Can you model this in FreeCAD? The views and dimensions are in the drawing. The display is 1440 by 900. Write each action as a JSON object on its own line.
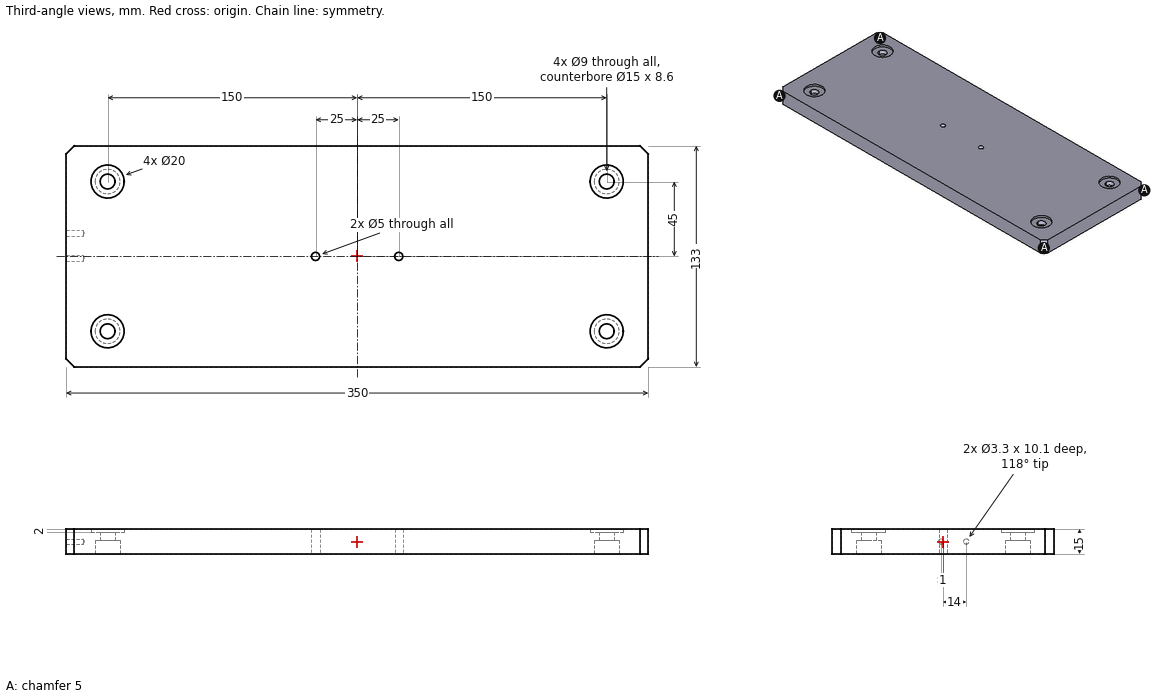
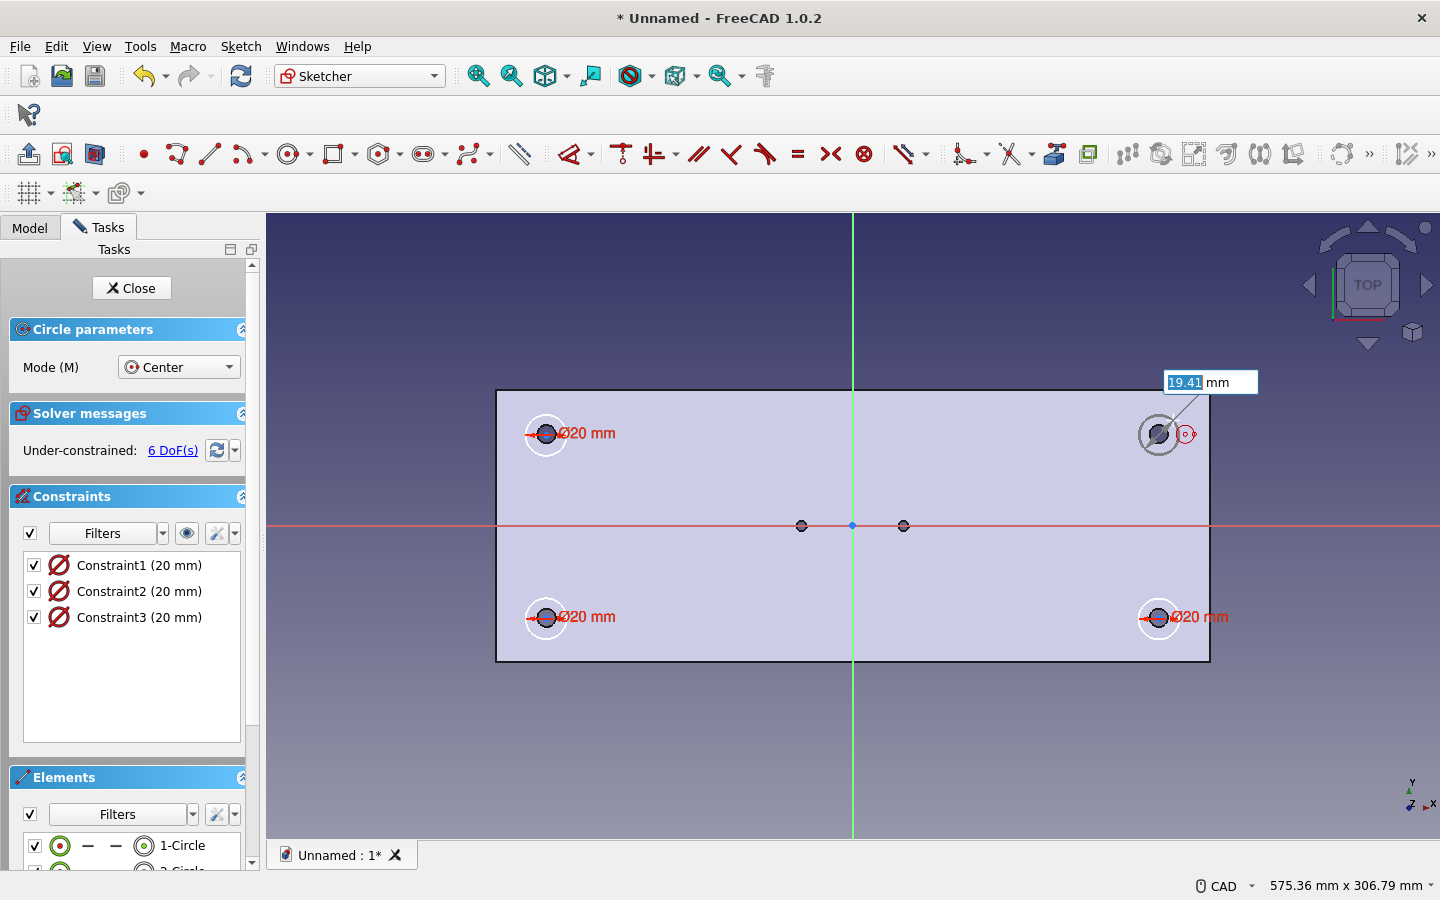
{"action": "type", "text": "20"}
{"action": "key", "text": "Return"}
{"action": "key", "text": "Escape"}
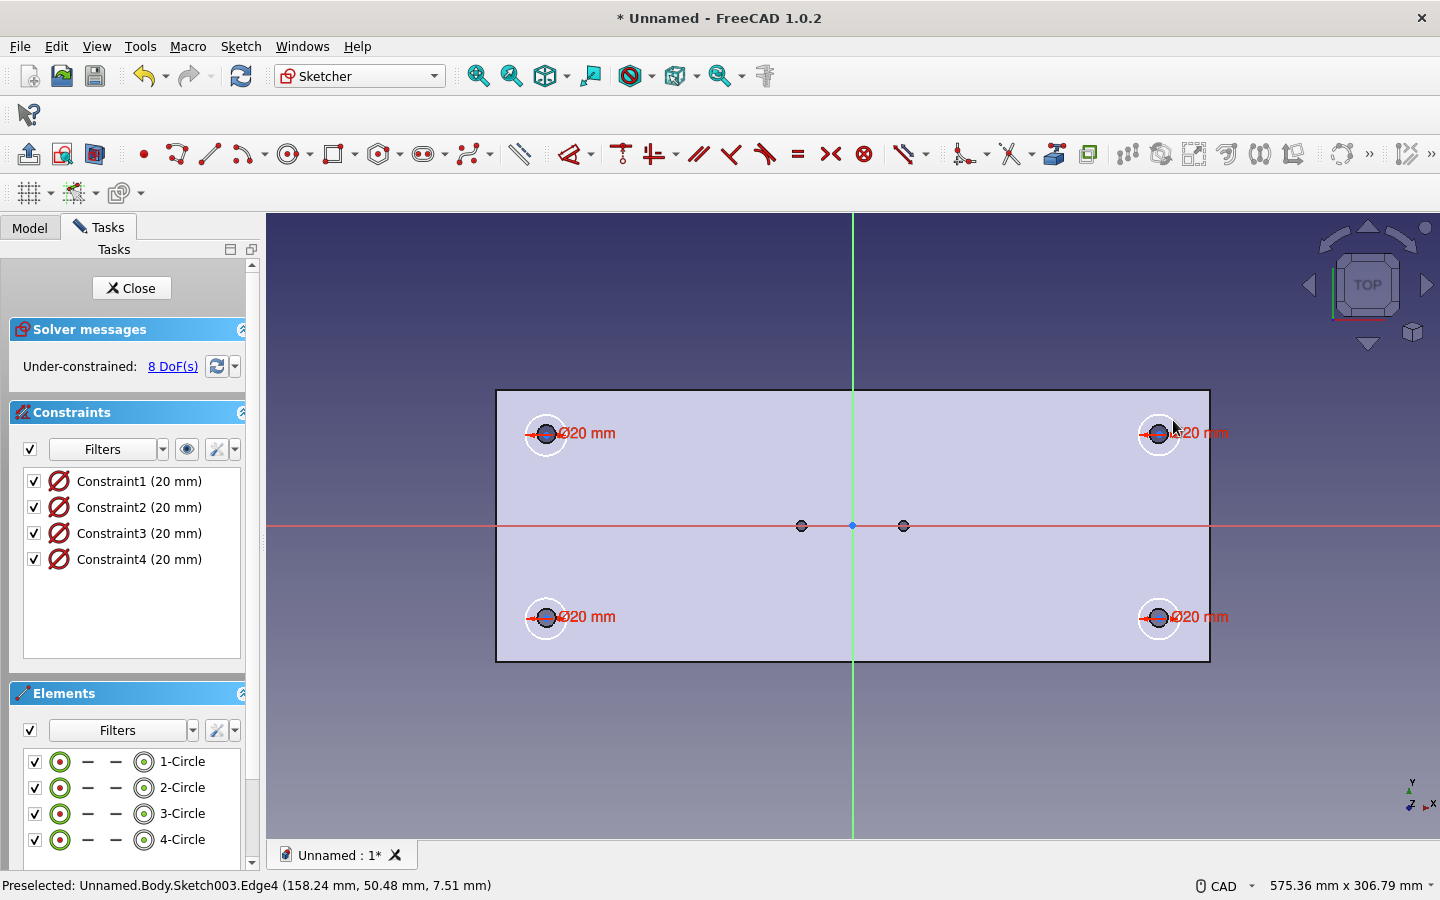
{"action": "left_click", "coordinate": [546, 435]}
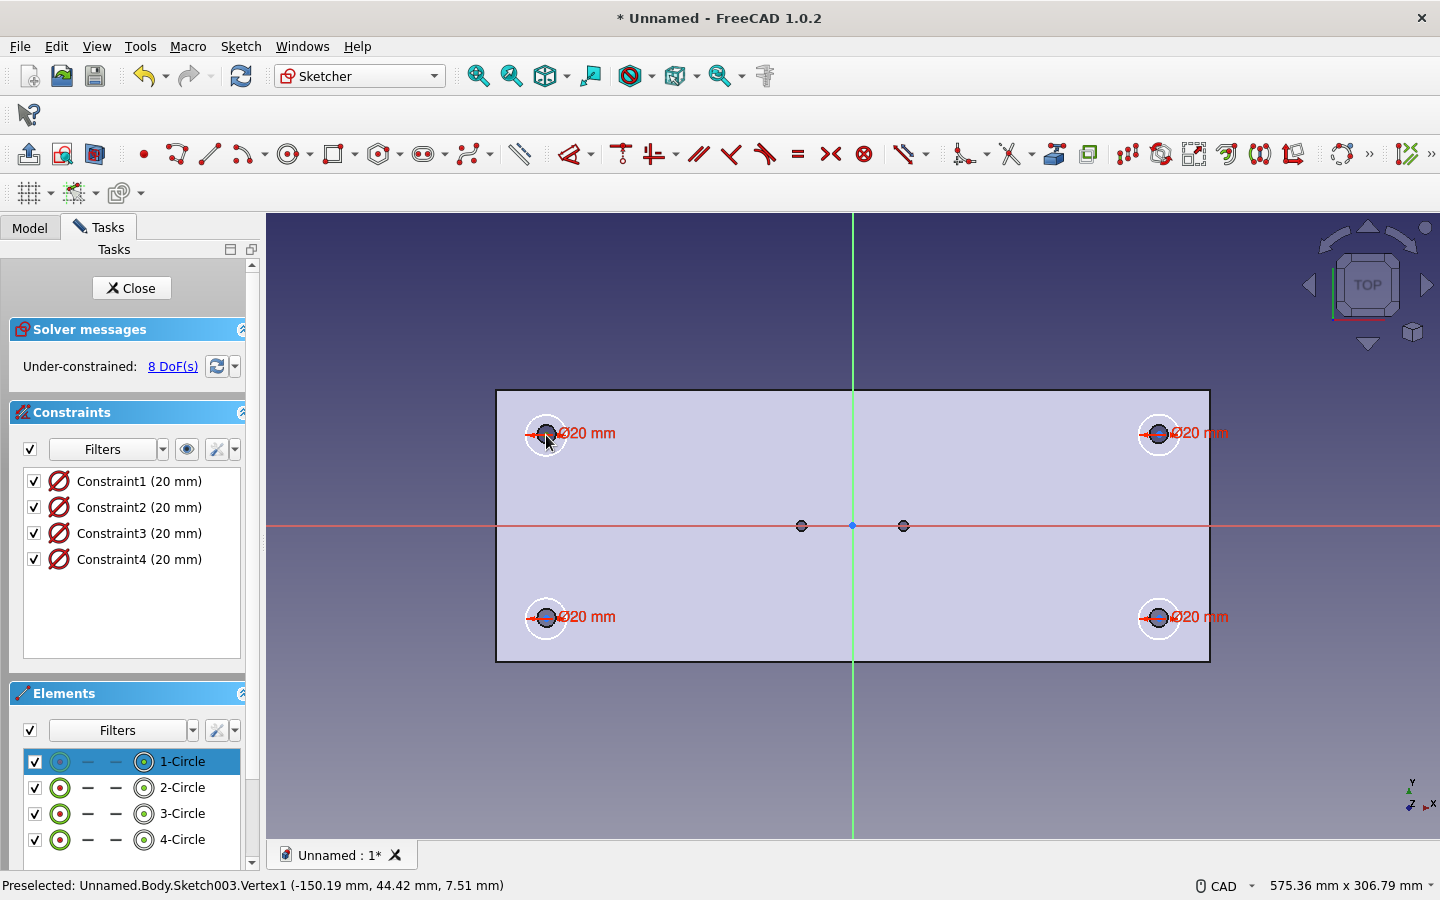
{"action": "left_click", "coordinate": [546, 619]}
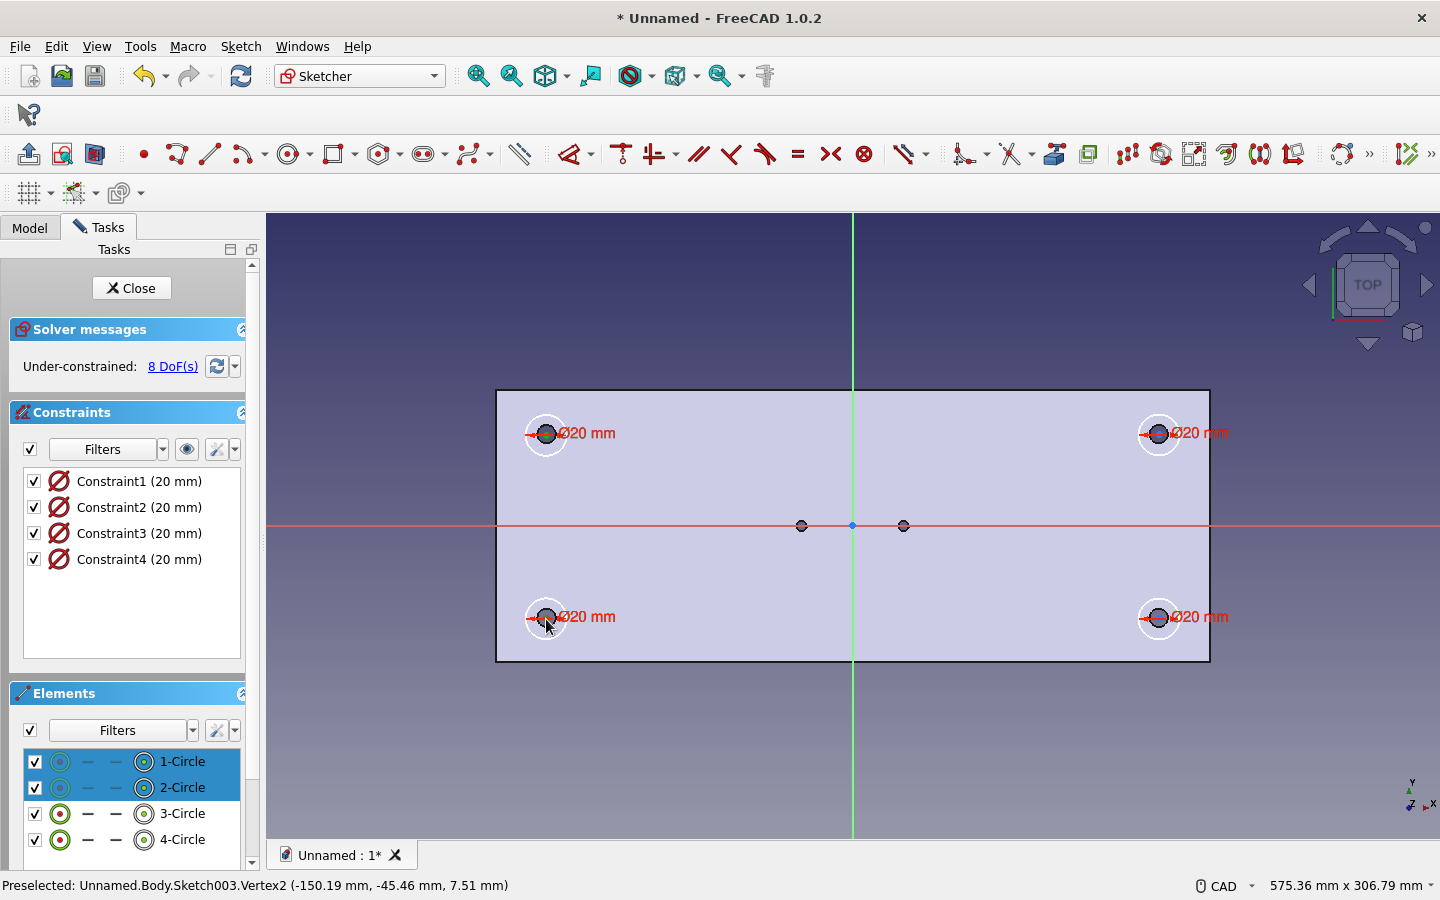
{"action": "left_click", "coordinate": [364, 526]}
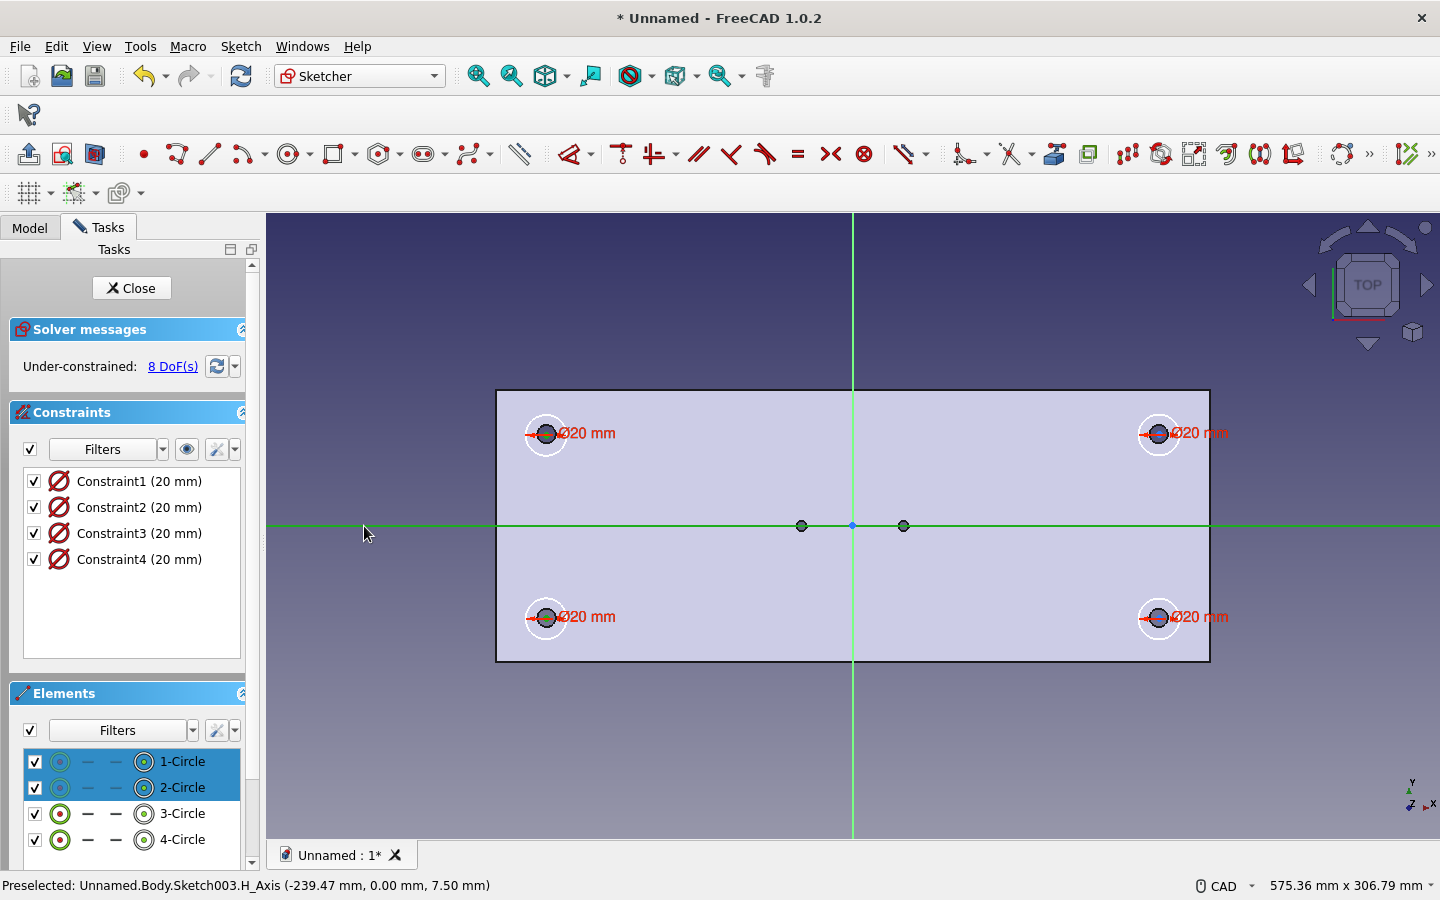
{"action": "key", "text": "s"}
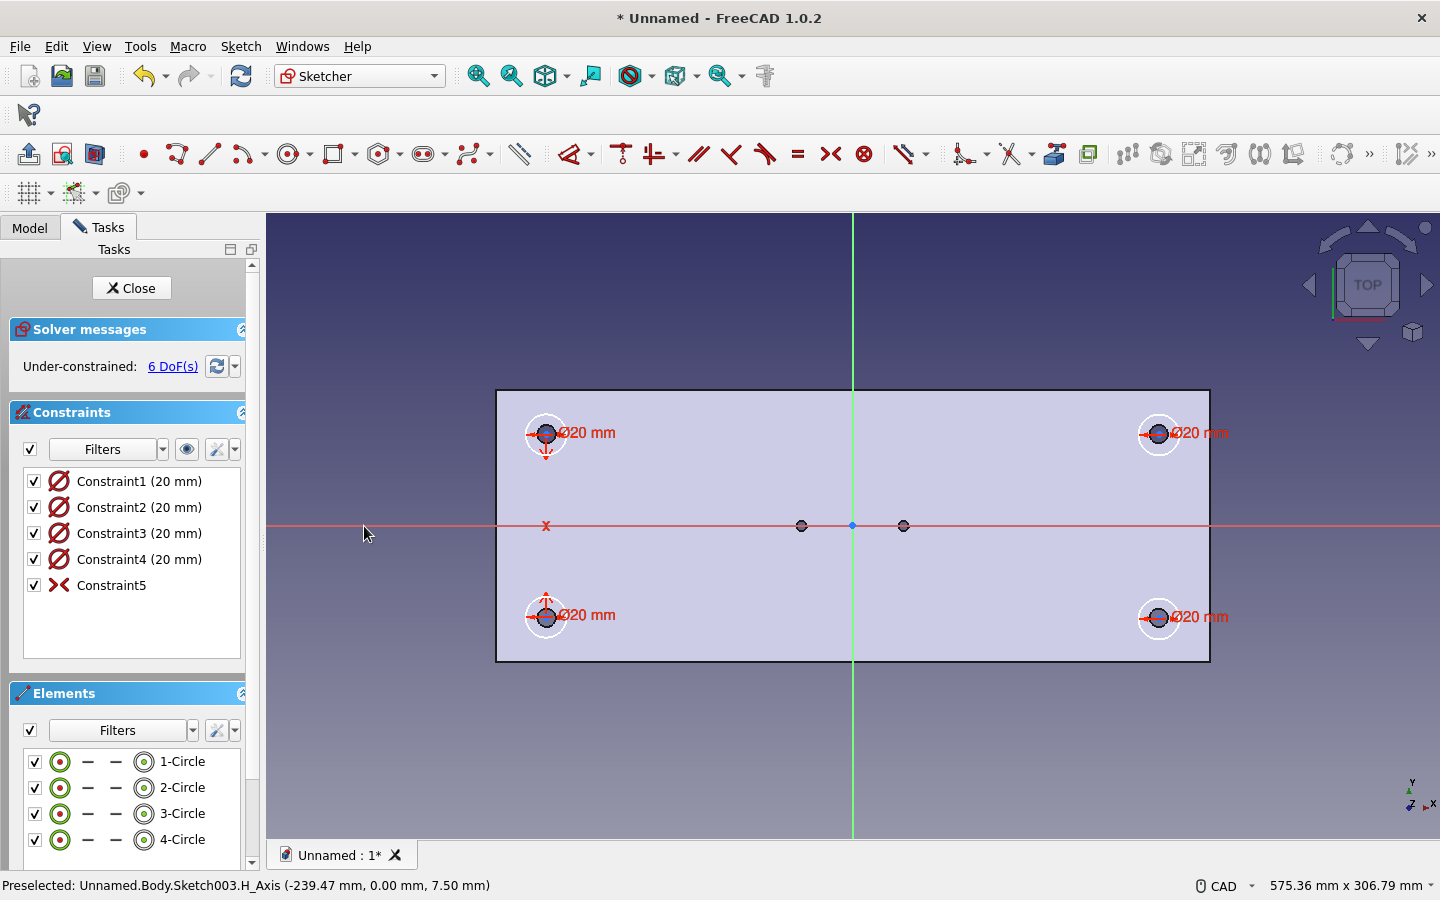
{"action": "left_click", "coordinate": [546, 617]}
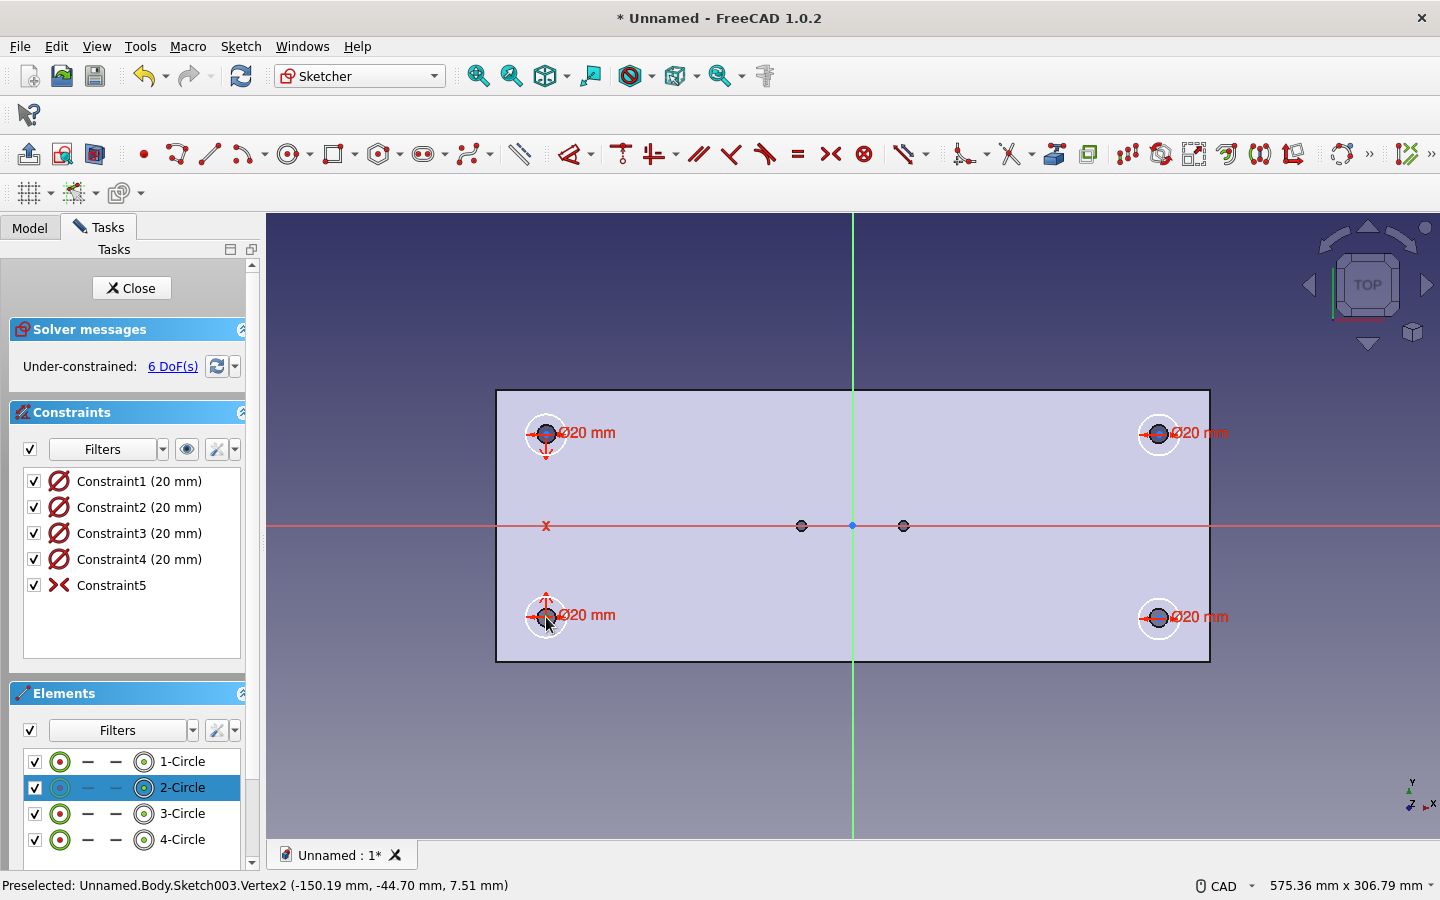
{"action": "left_click", "coordinate": [1159, 619]}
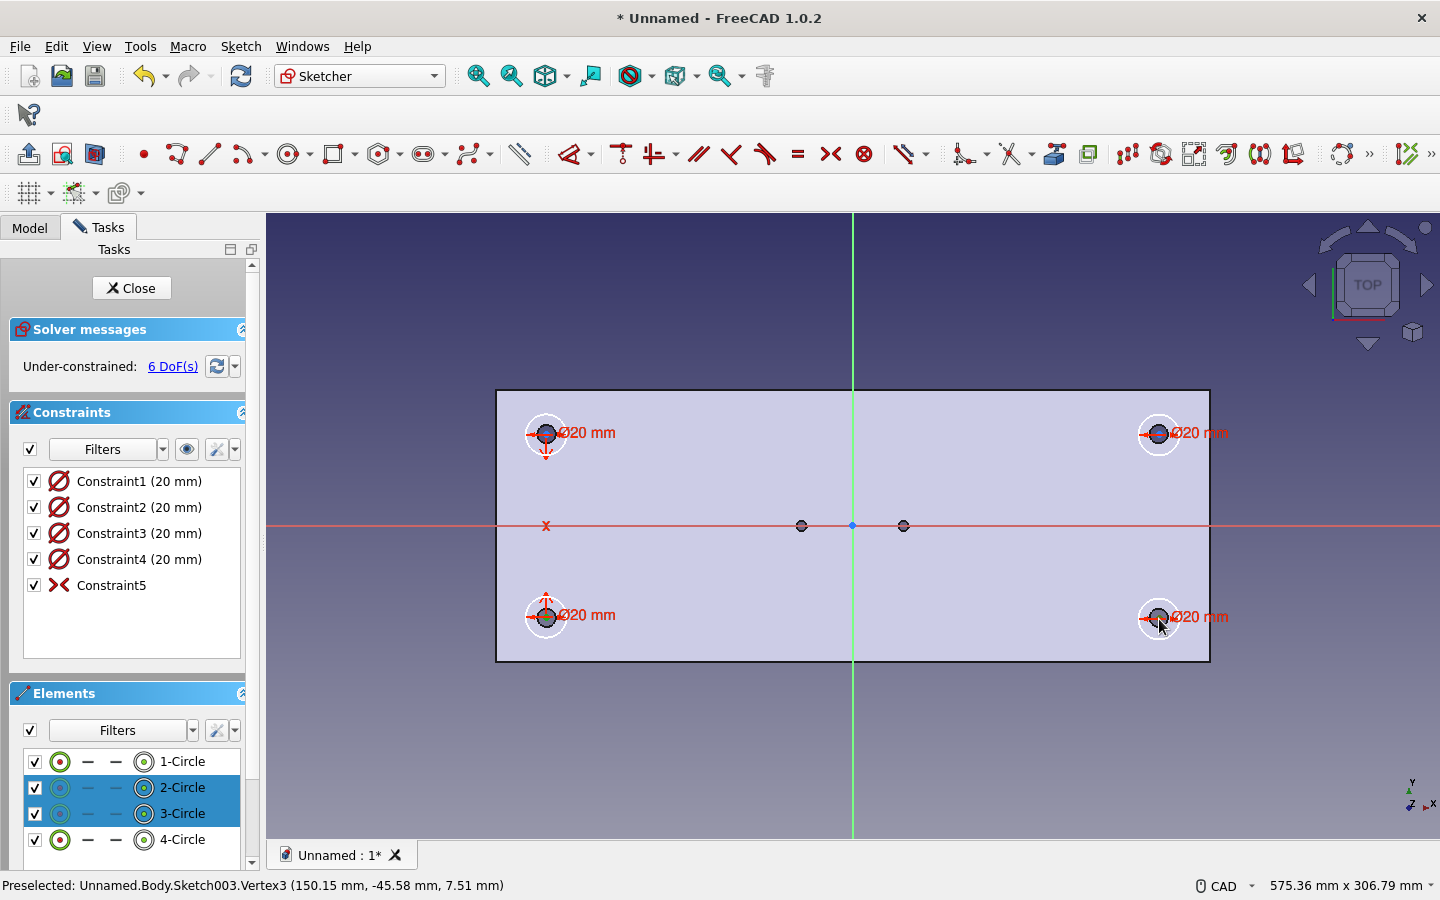
{"action": "left_click", "coordinate": [853, 770]}